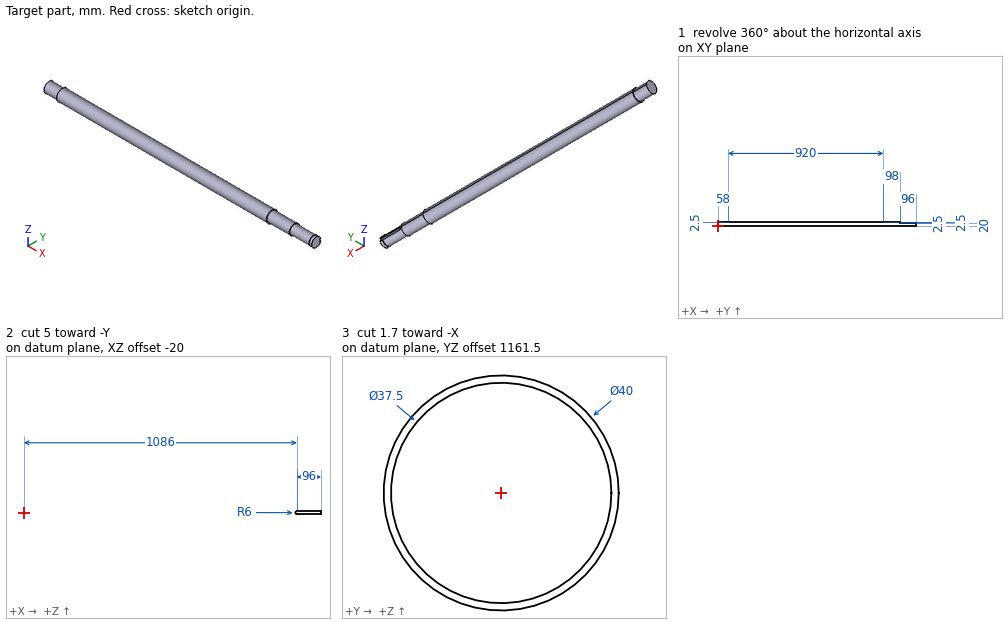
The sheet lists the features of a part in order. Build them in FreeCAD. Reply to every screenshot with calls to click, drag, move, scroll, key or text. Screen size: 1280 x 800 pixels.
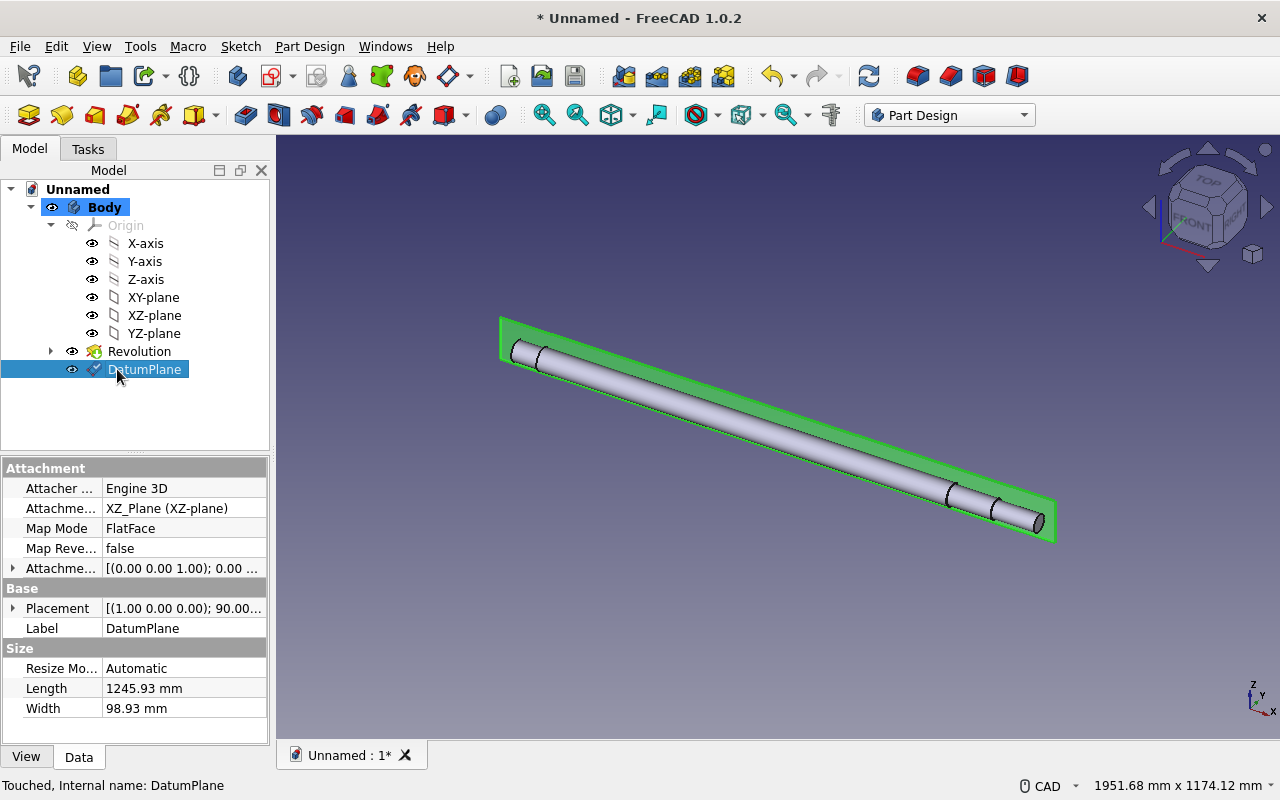
click(270, 76)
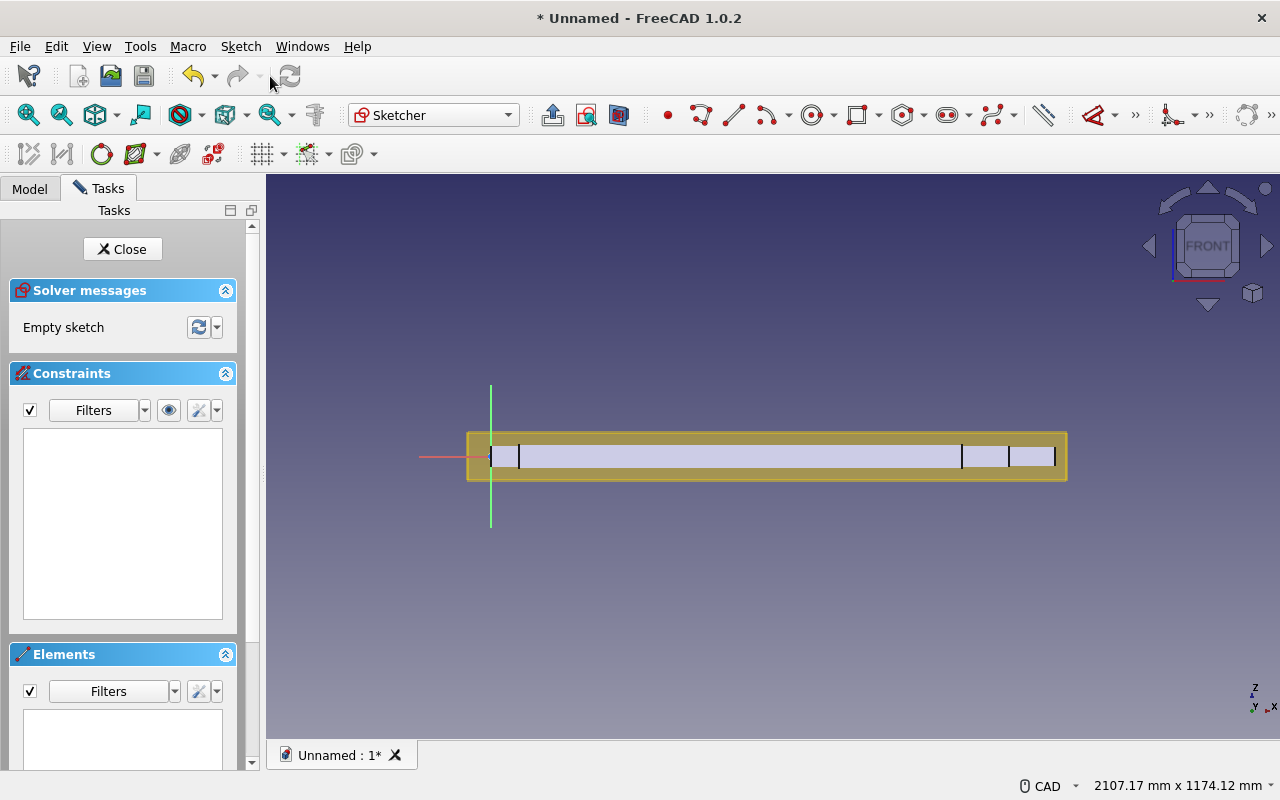
click(619, 116)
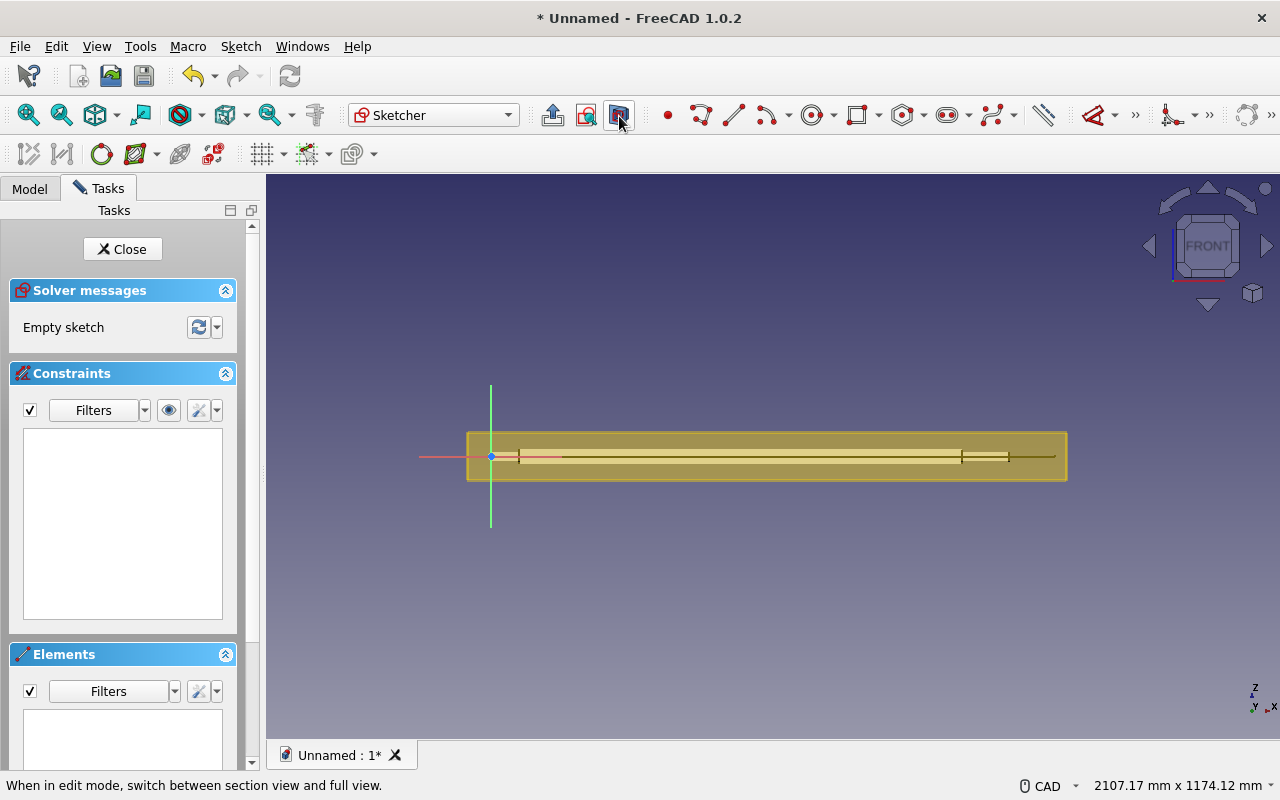
scroll(1068, 457, up, 12)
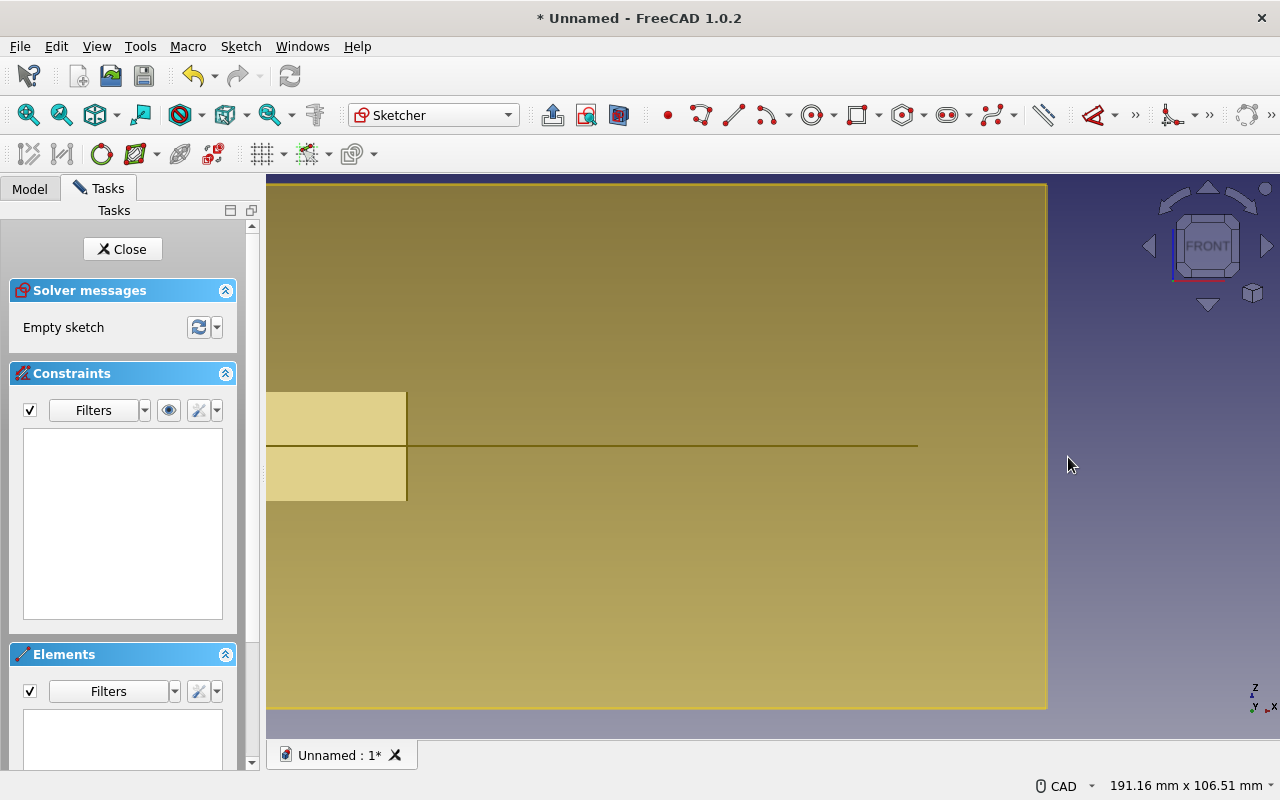
click(701, 116)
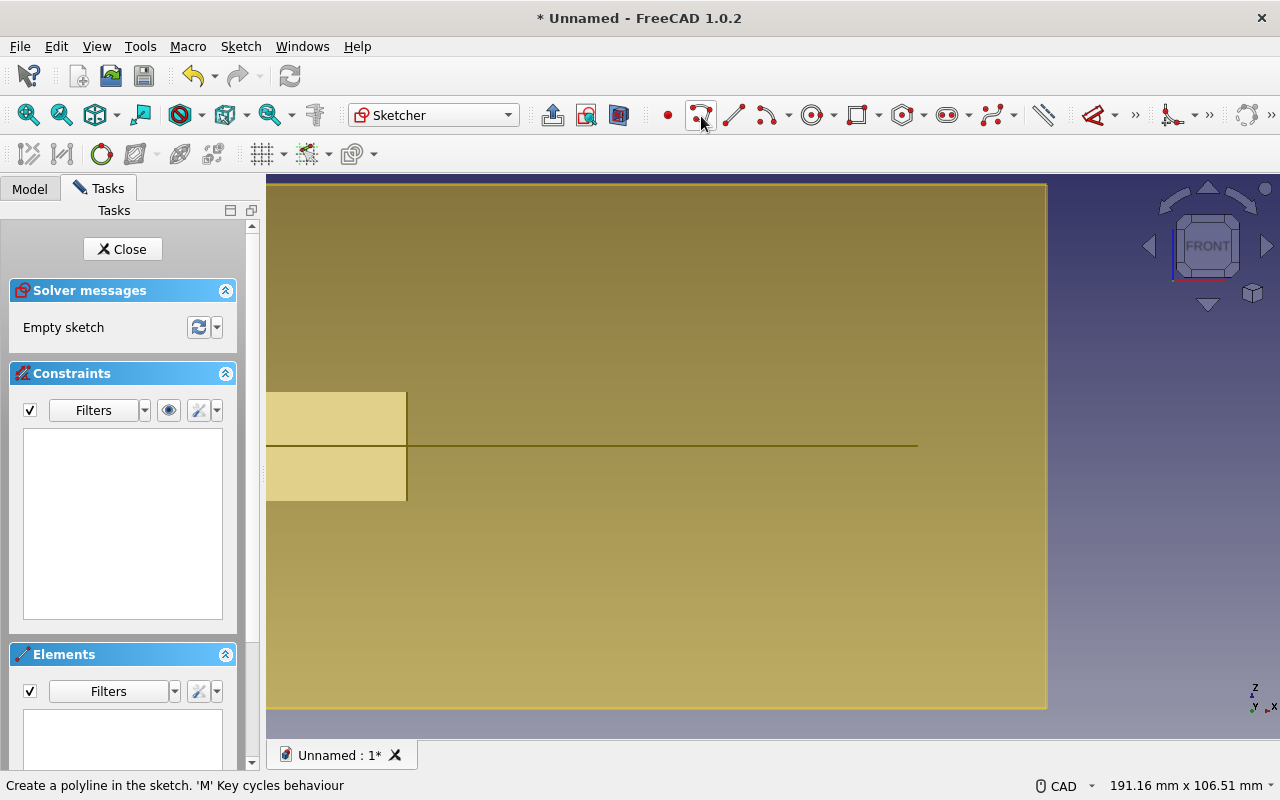
click(460, 415)
click(970, 415)
click(970, 478)
click(460, 478)
right_click(460, 478)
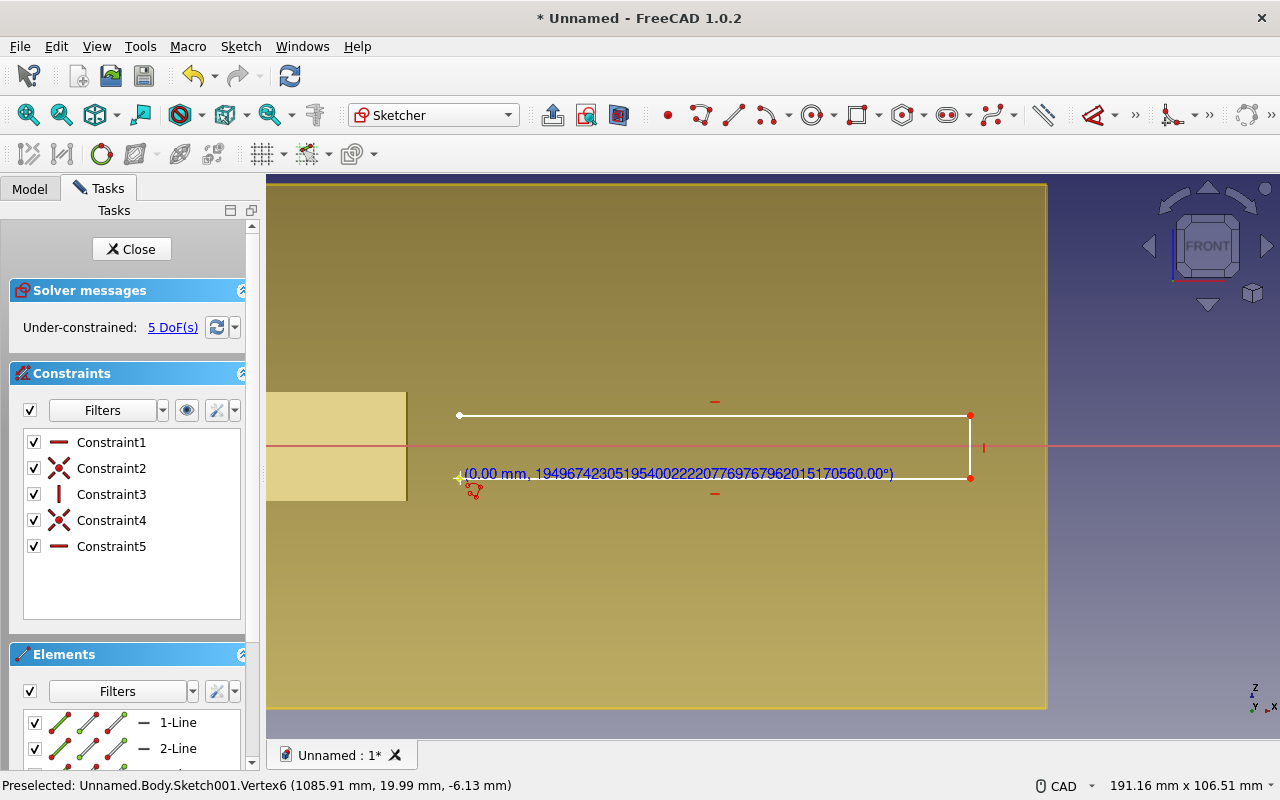
key(g)
key(3)
key(a)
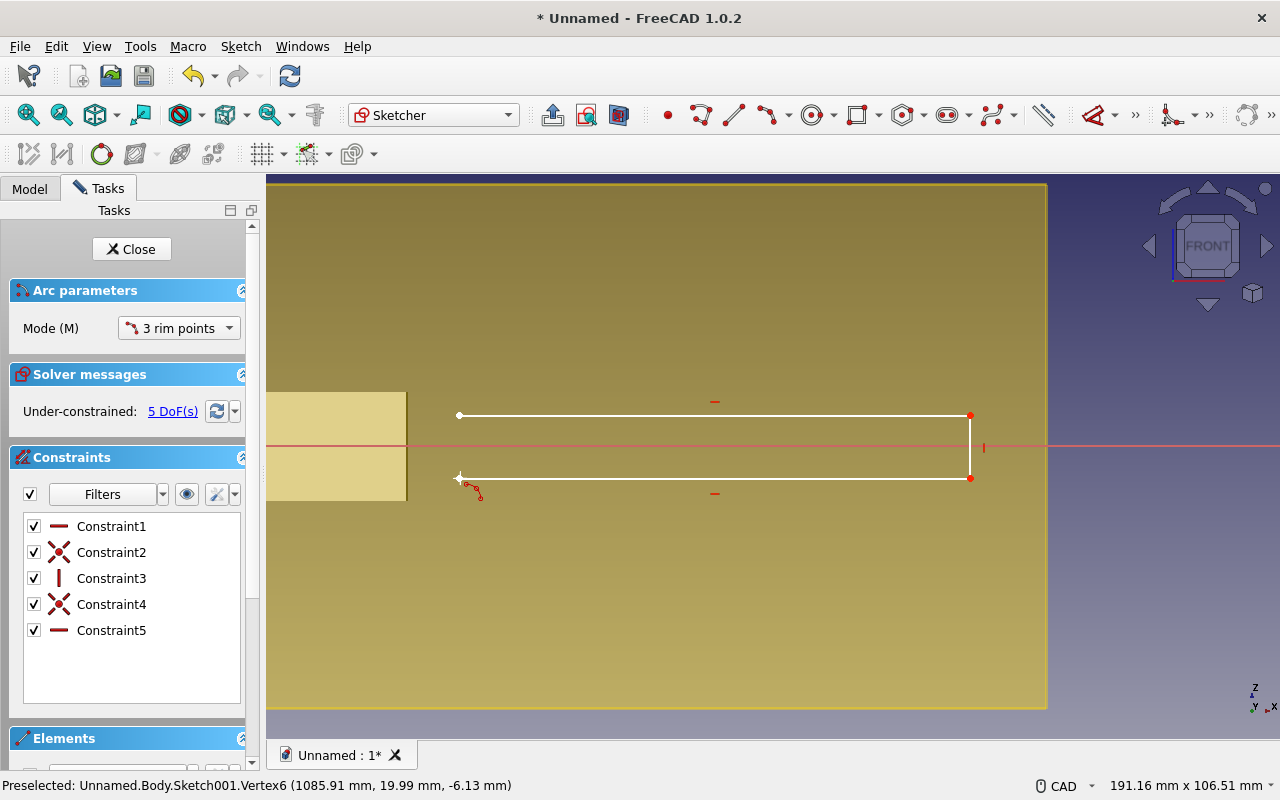
click(460, 479)
click(460, 416)
click(435, 428)
key(Escape)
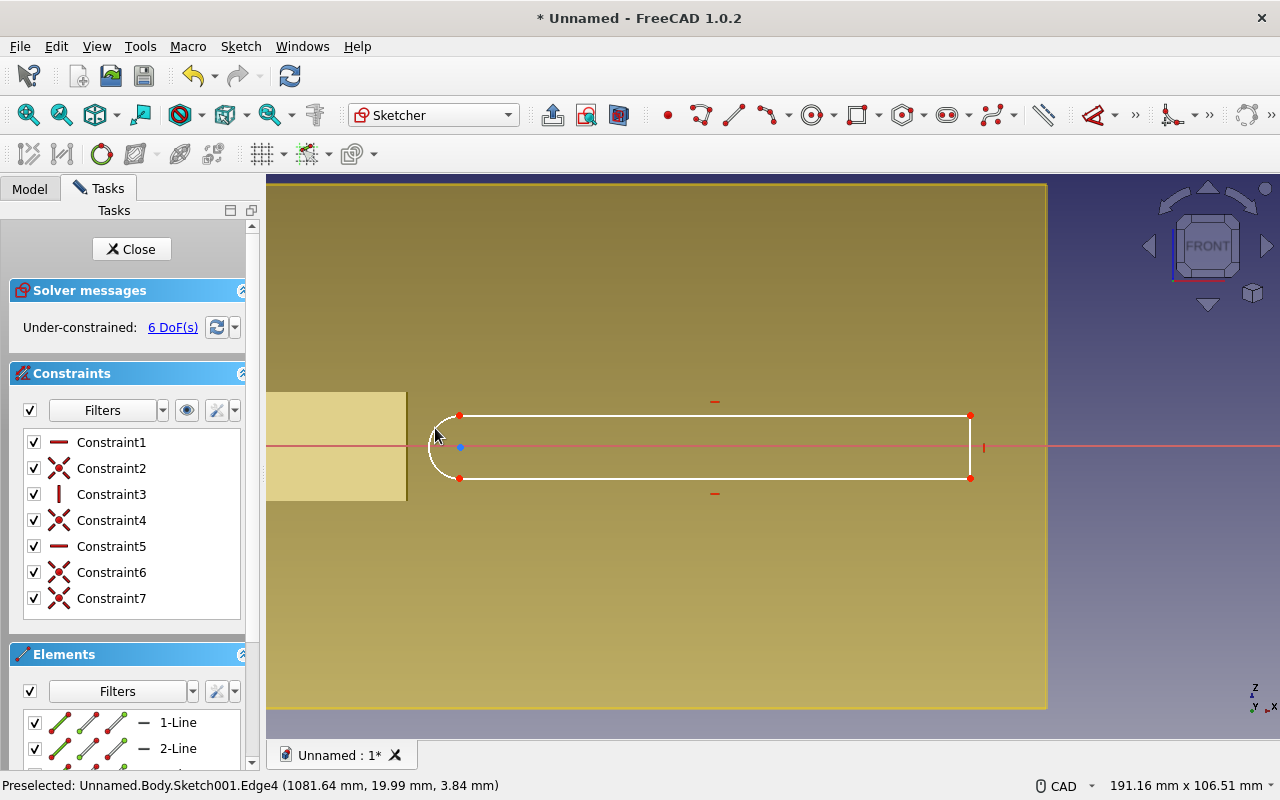
click(613, 416)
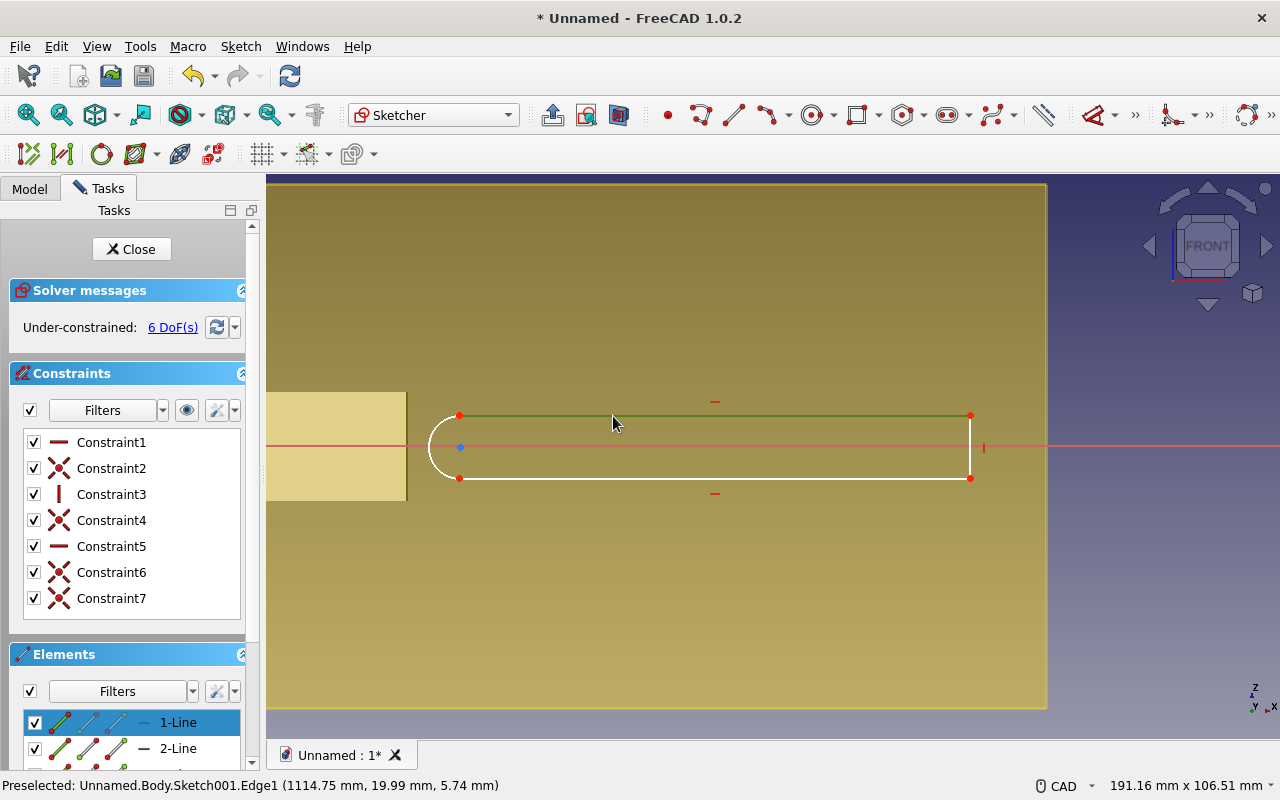
click(435, 429)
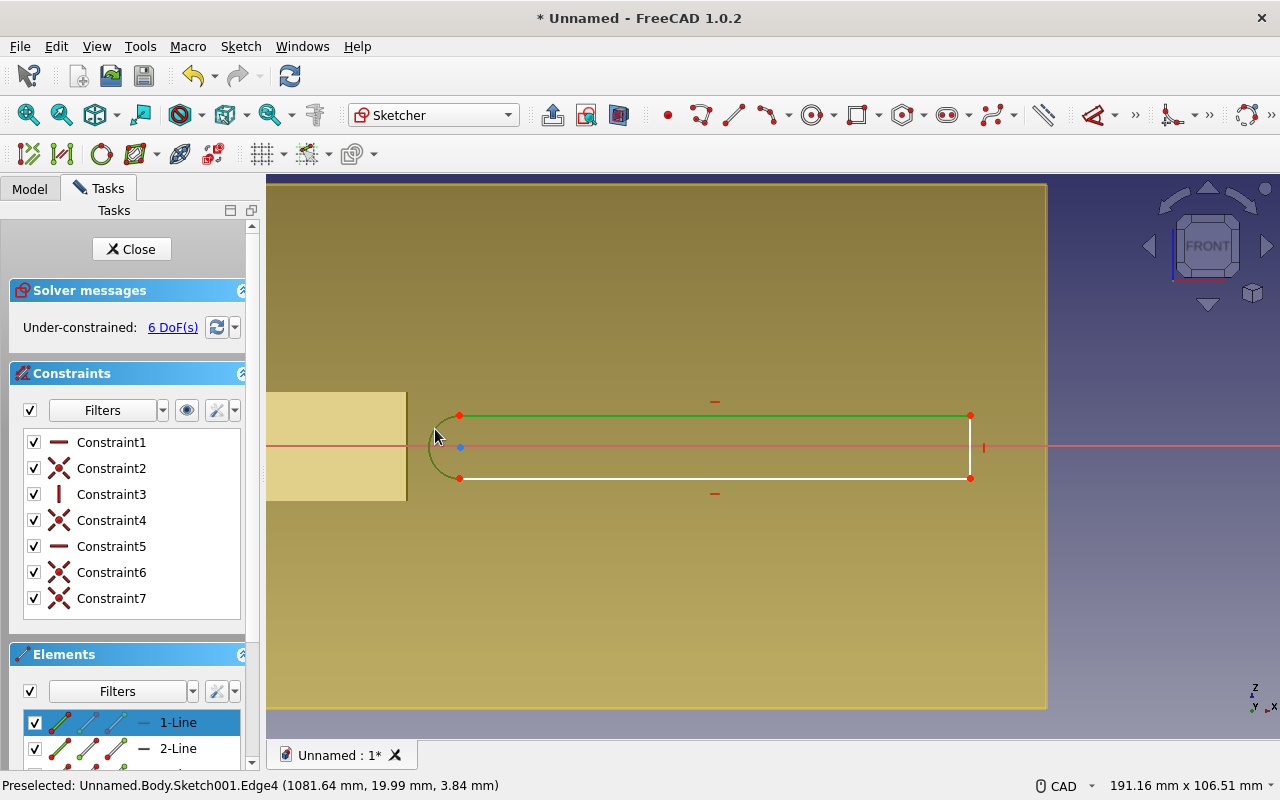
key(t)